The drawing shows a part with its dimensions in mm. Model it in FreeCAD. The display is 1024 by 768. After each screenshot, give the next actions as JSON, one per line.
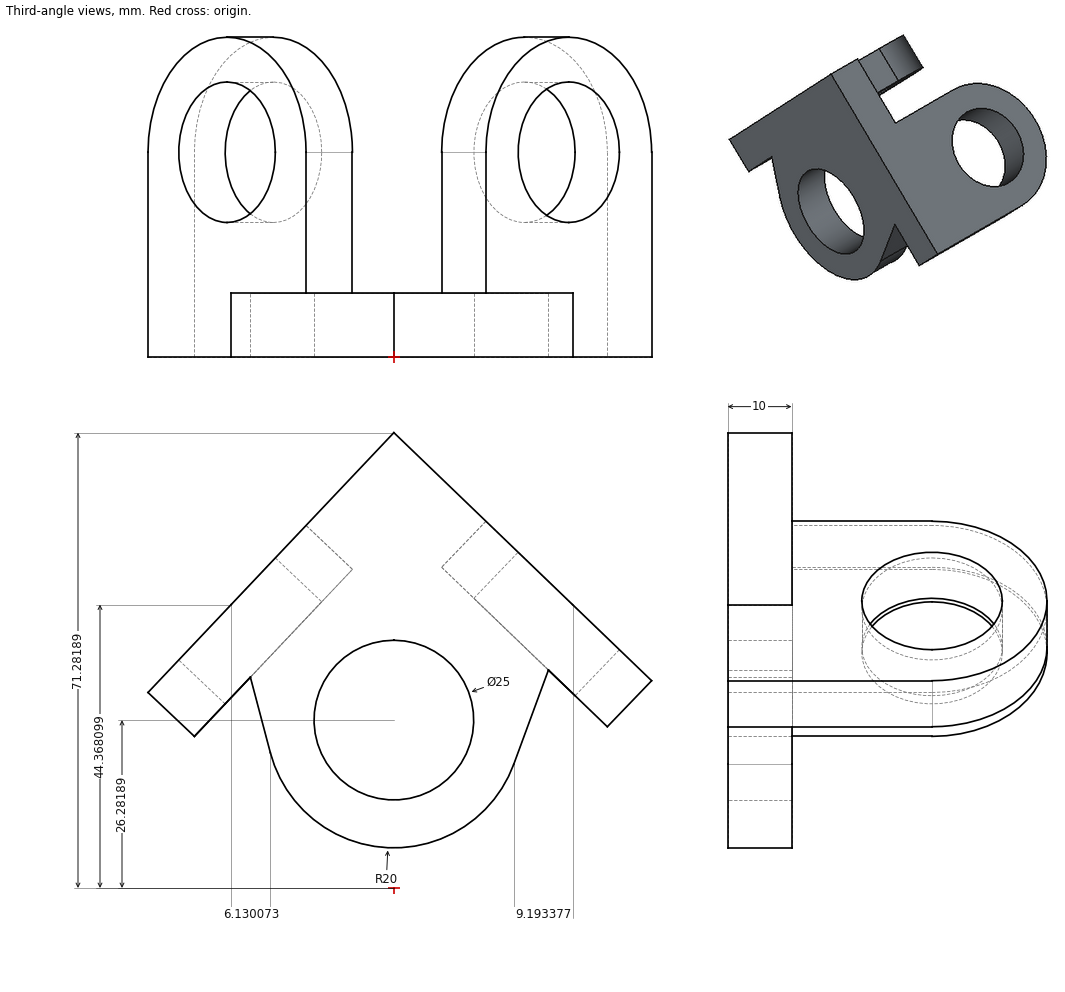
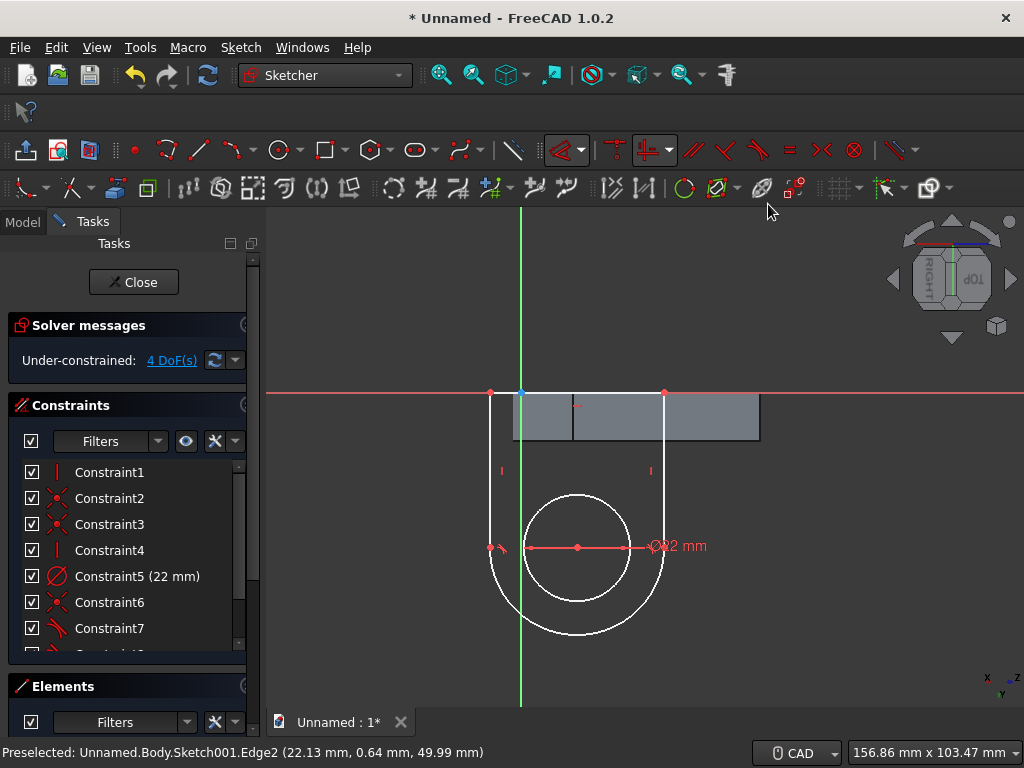
{"action": "left_click", "coordinate": [628, 618]}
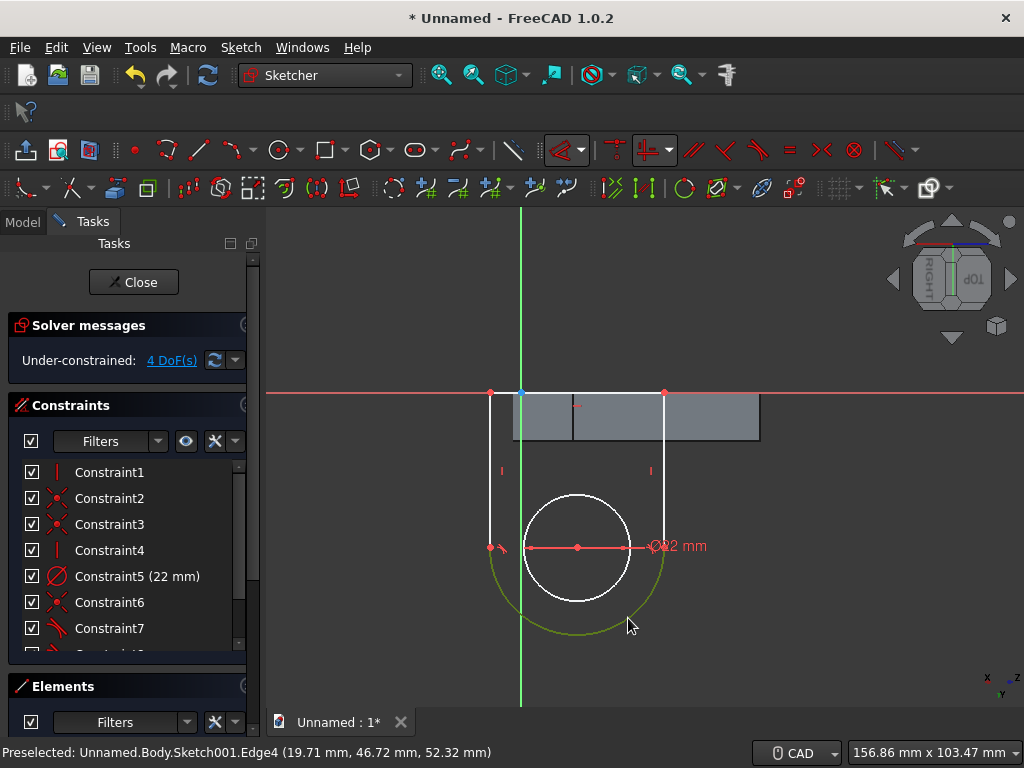
{"action": "left_click", "coordinate": [584, 150]}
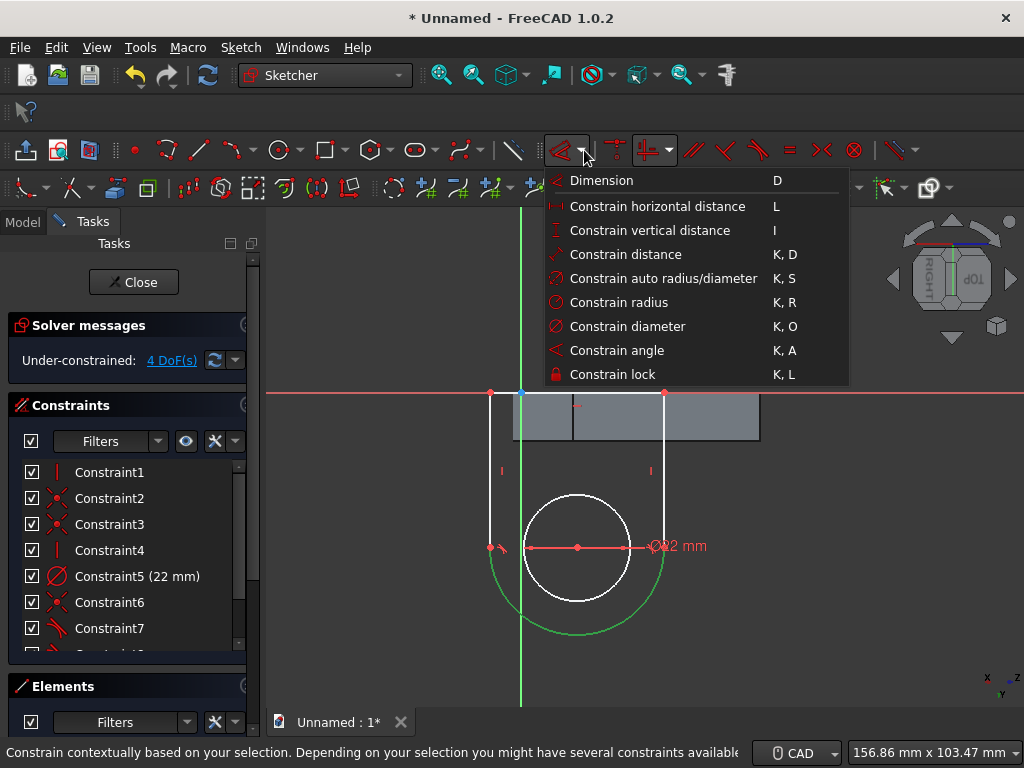
{"action": "left_click", "coordinate": [697, 302]}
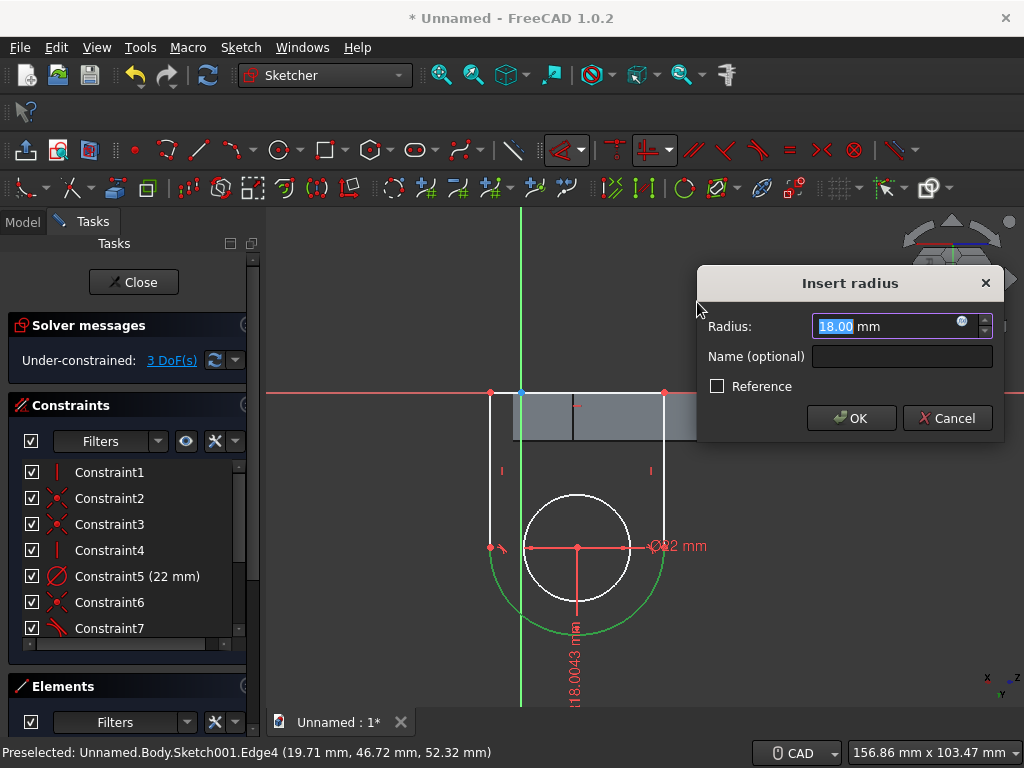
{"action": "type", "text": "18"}
{"action": "key", "text": "Return"}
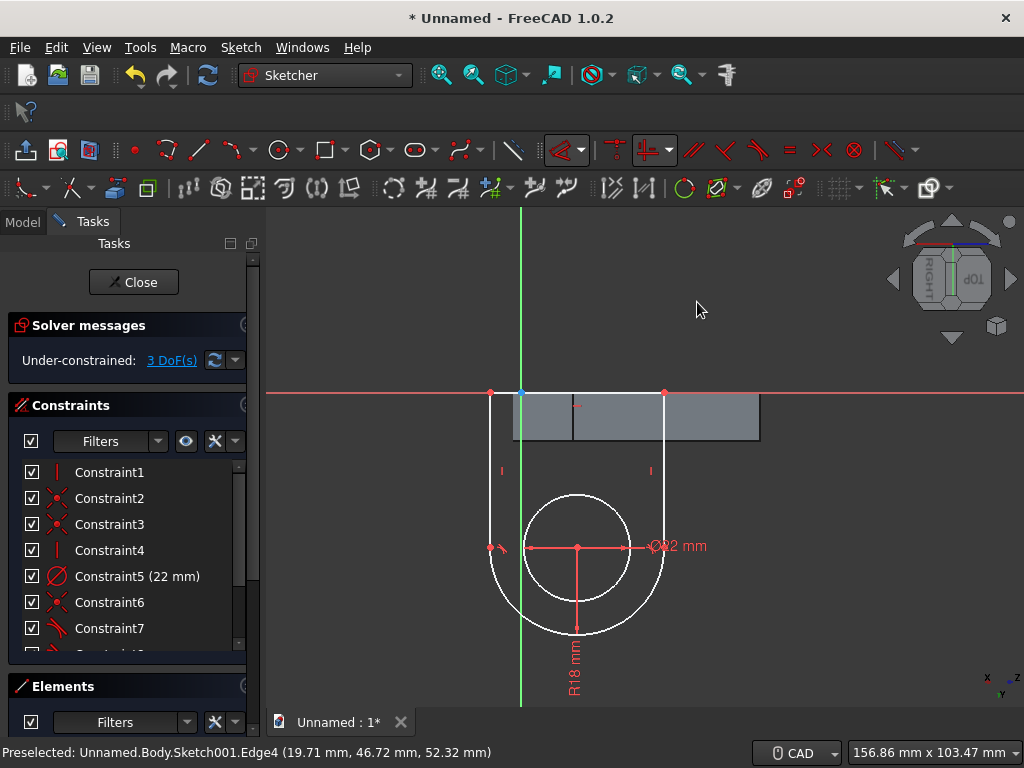
{"action": "left_click", "coordinate": [664, 393]}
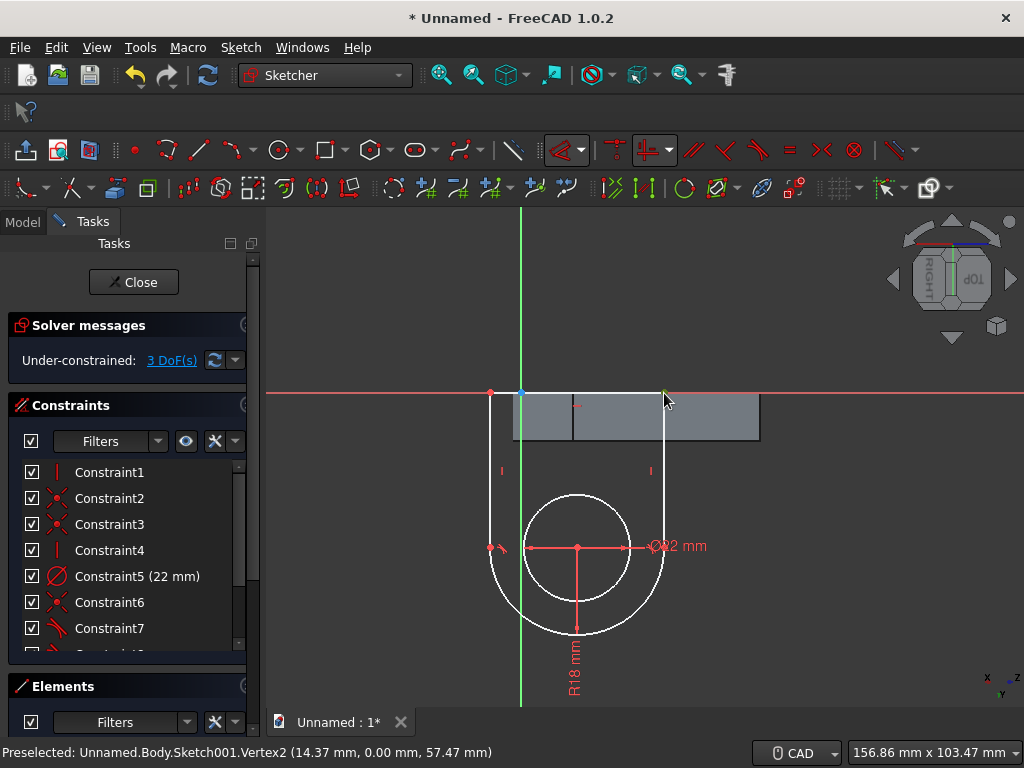
{"action": "left_click", "coordinate": [334, 393]}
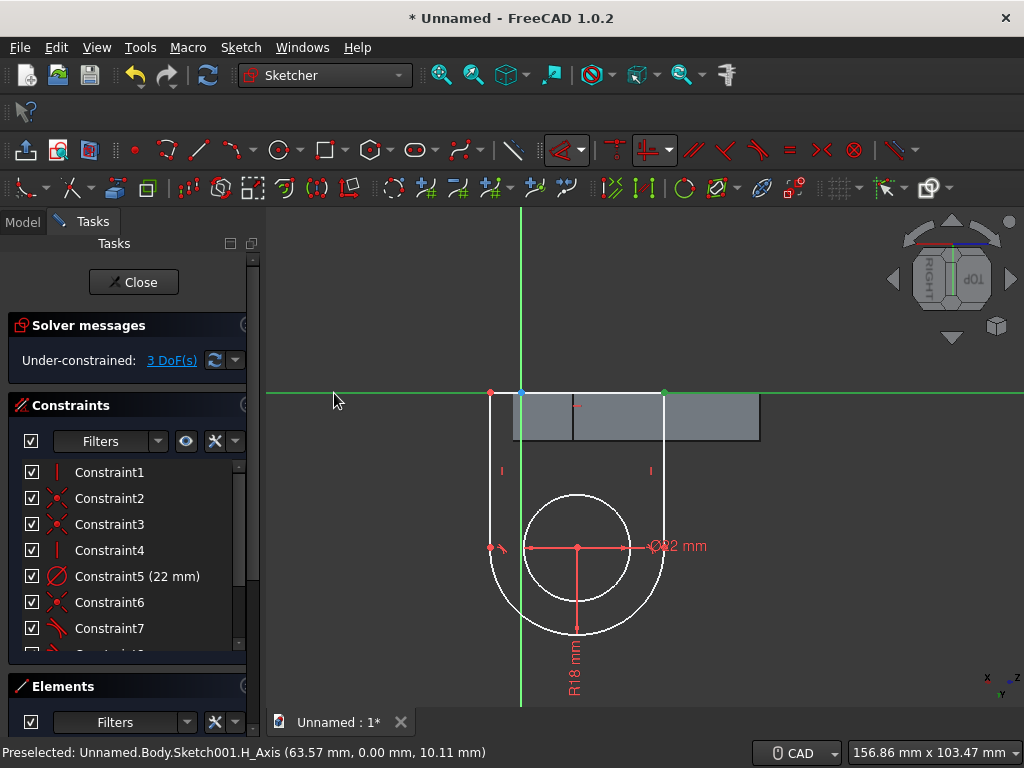
{"action": "left_click", "coordinate": [616, 150]}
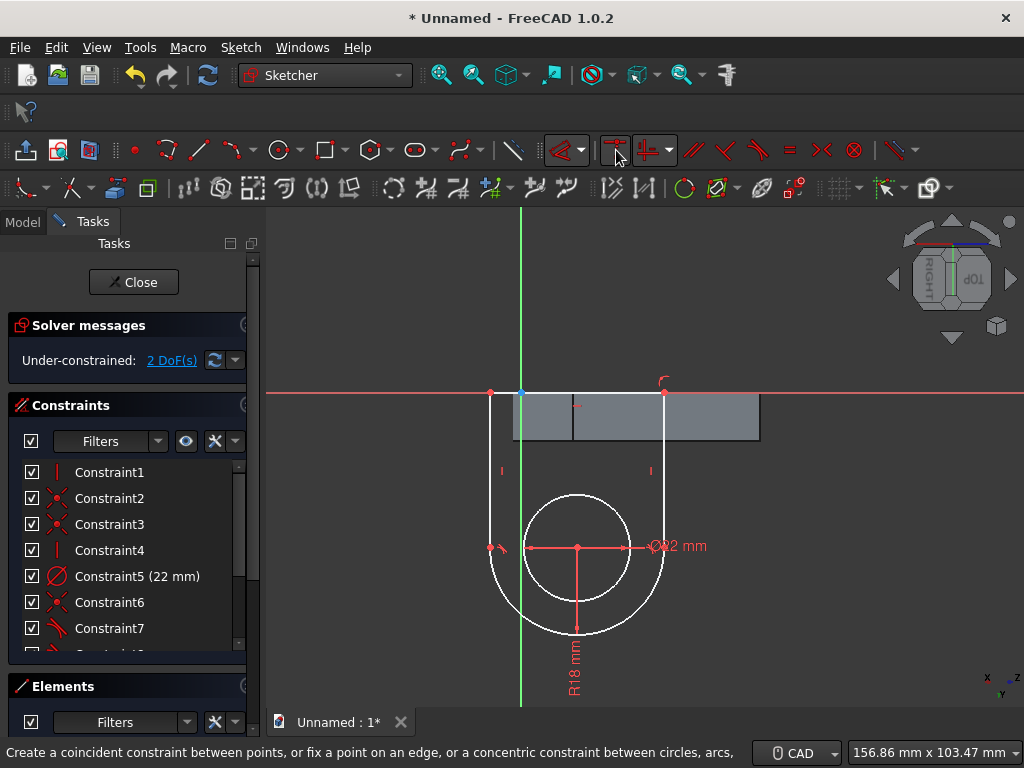
{"action": "left_click", "coordinate": [664, 501]}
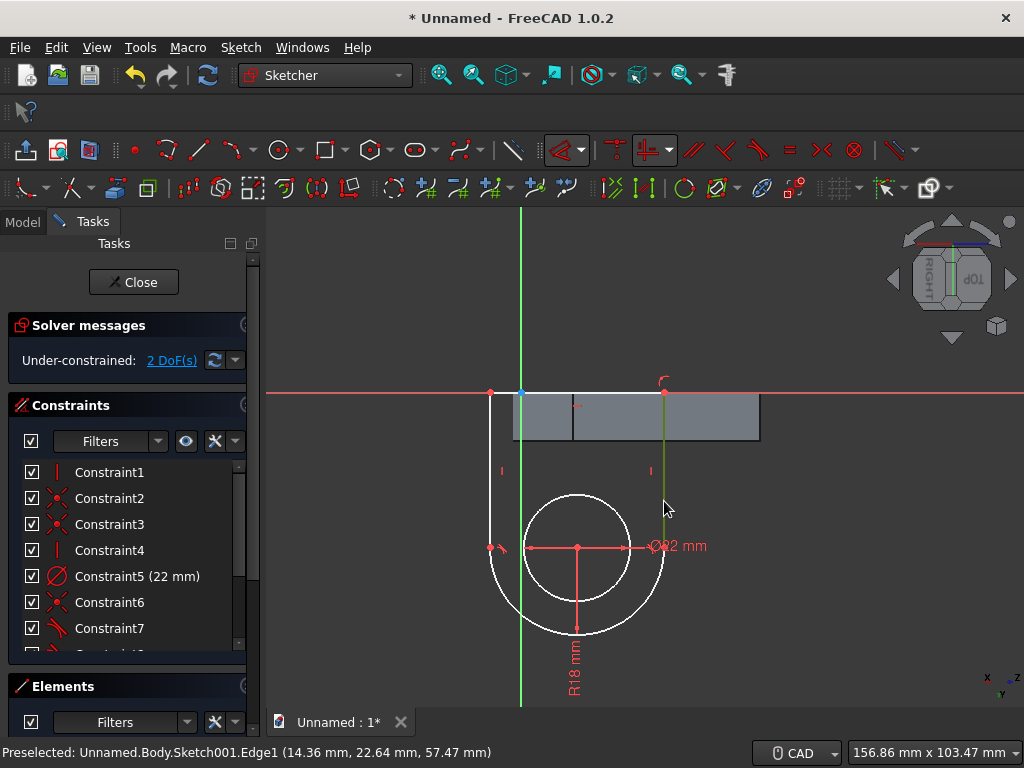
{"action": "key", "text": "i"}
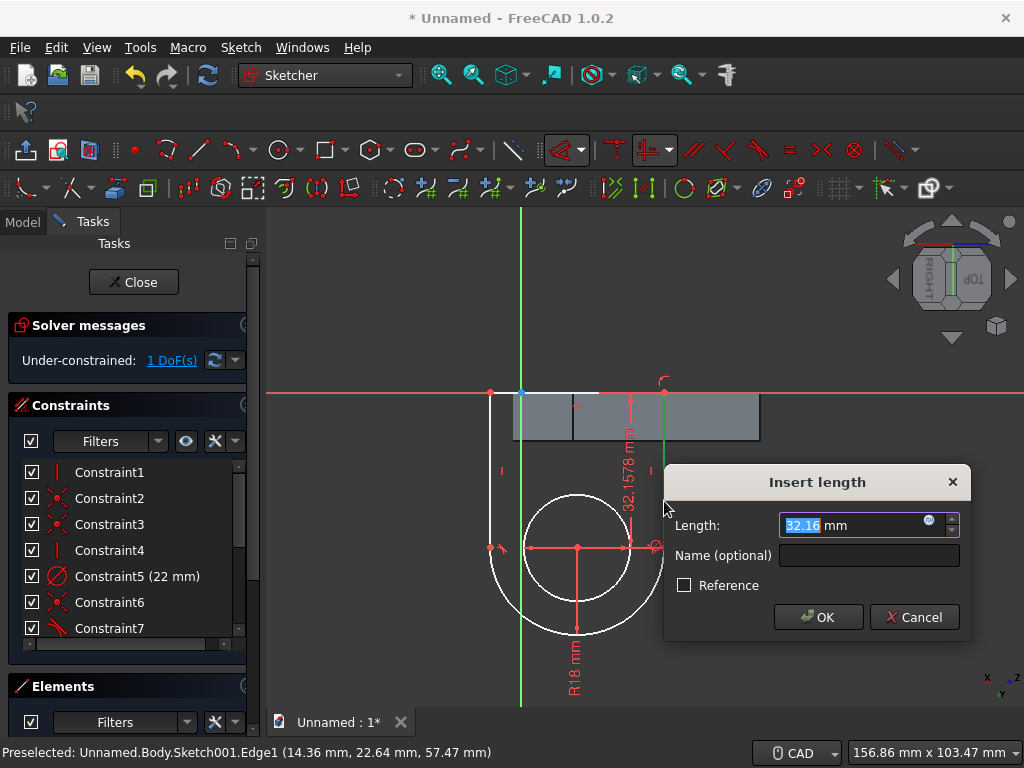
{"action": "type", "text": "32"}
{"action": "key", "text": "Return"}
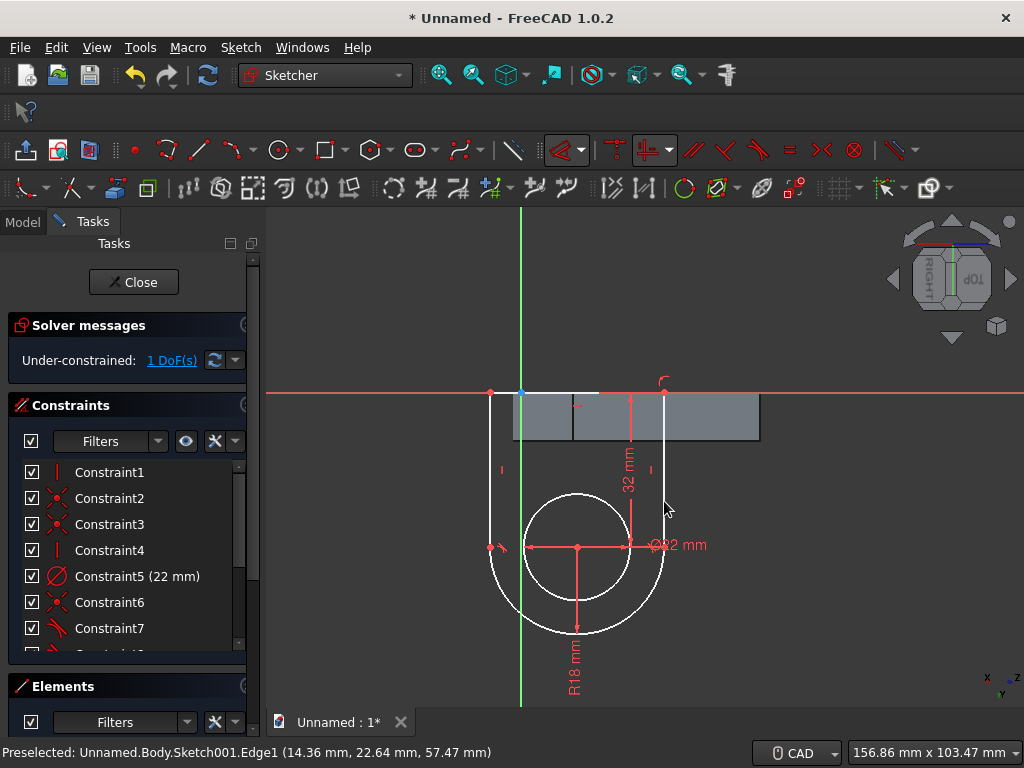
{"action": "scroll", "coordinate": [490, 393], "scroll_direction": "up", "scroll_amount": 2}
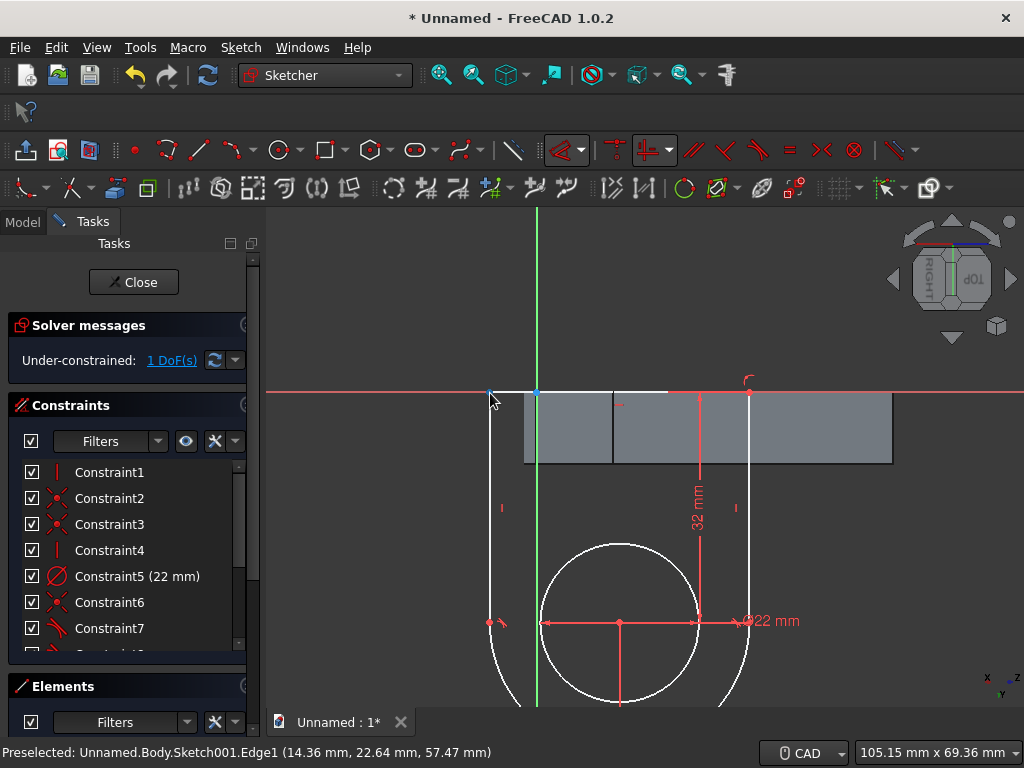
{"action": "left_click", "coordinate": [490, 392]}